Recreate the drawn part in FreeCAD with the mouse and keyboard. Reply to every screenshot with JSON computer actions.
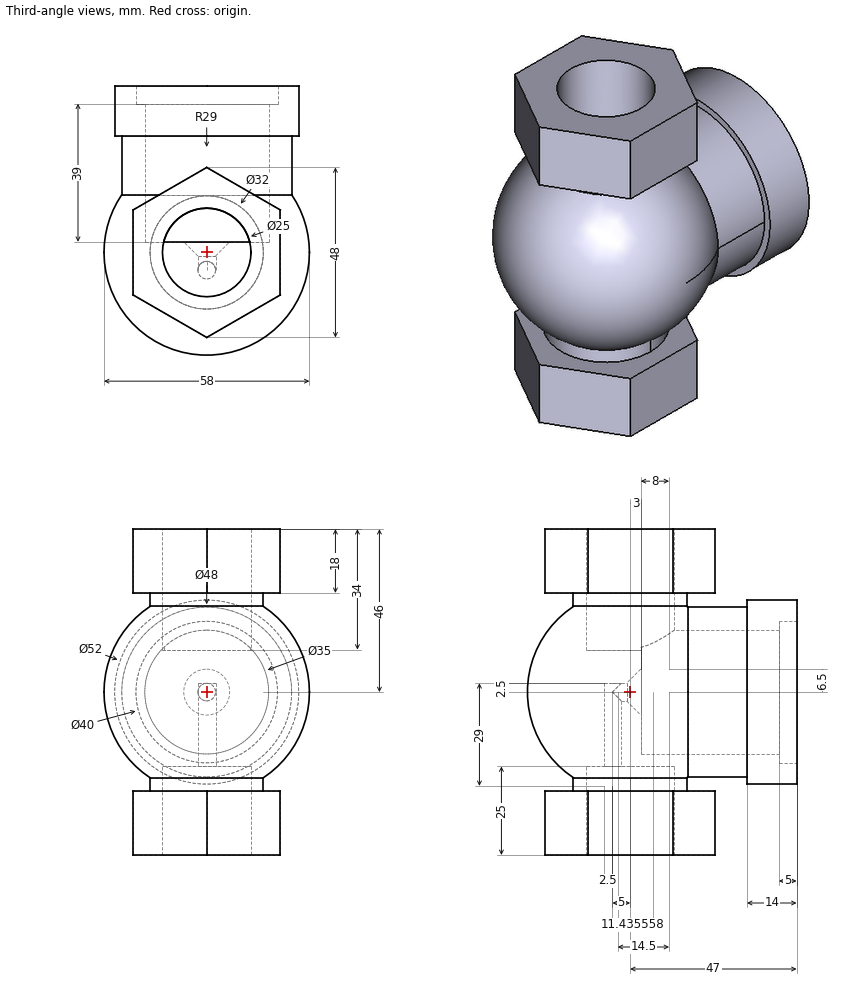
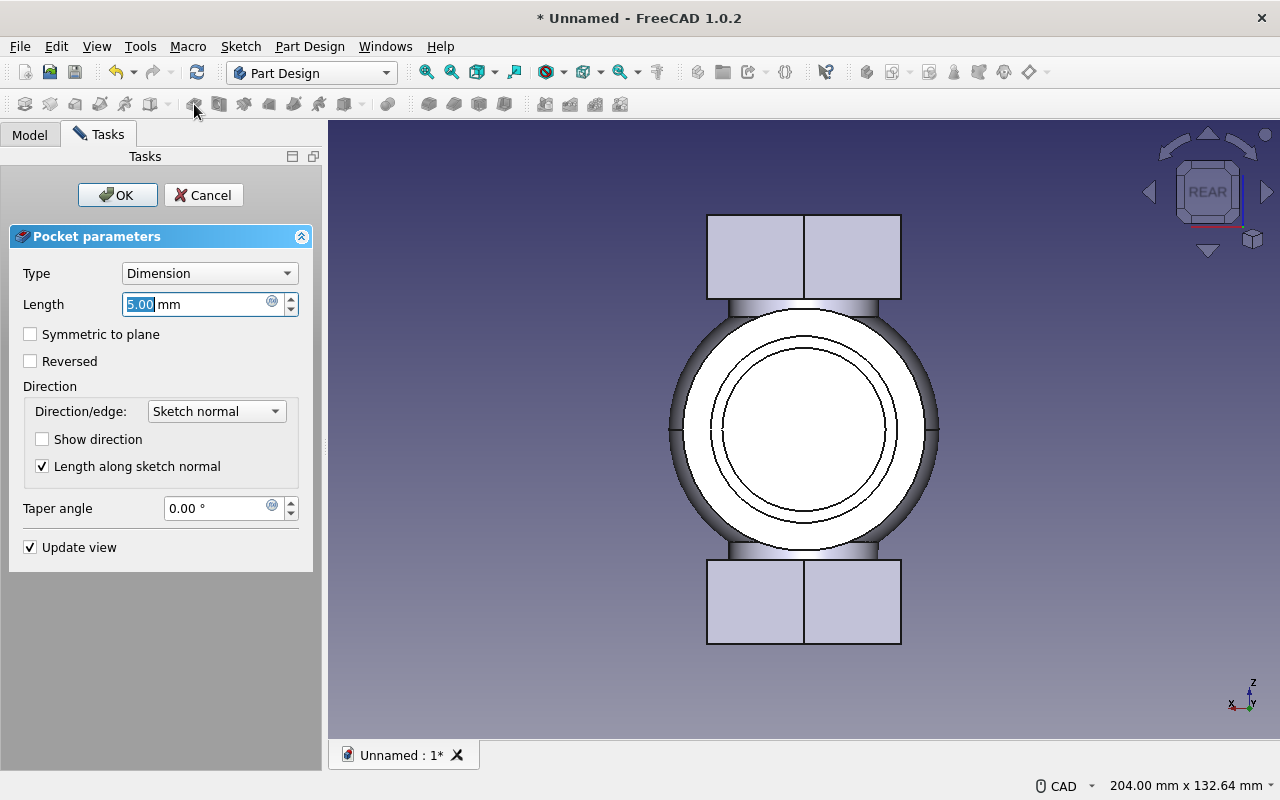
{"action": "type", "text": "39"}
{"action": "key", "text": "Tab"}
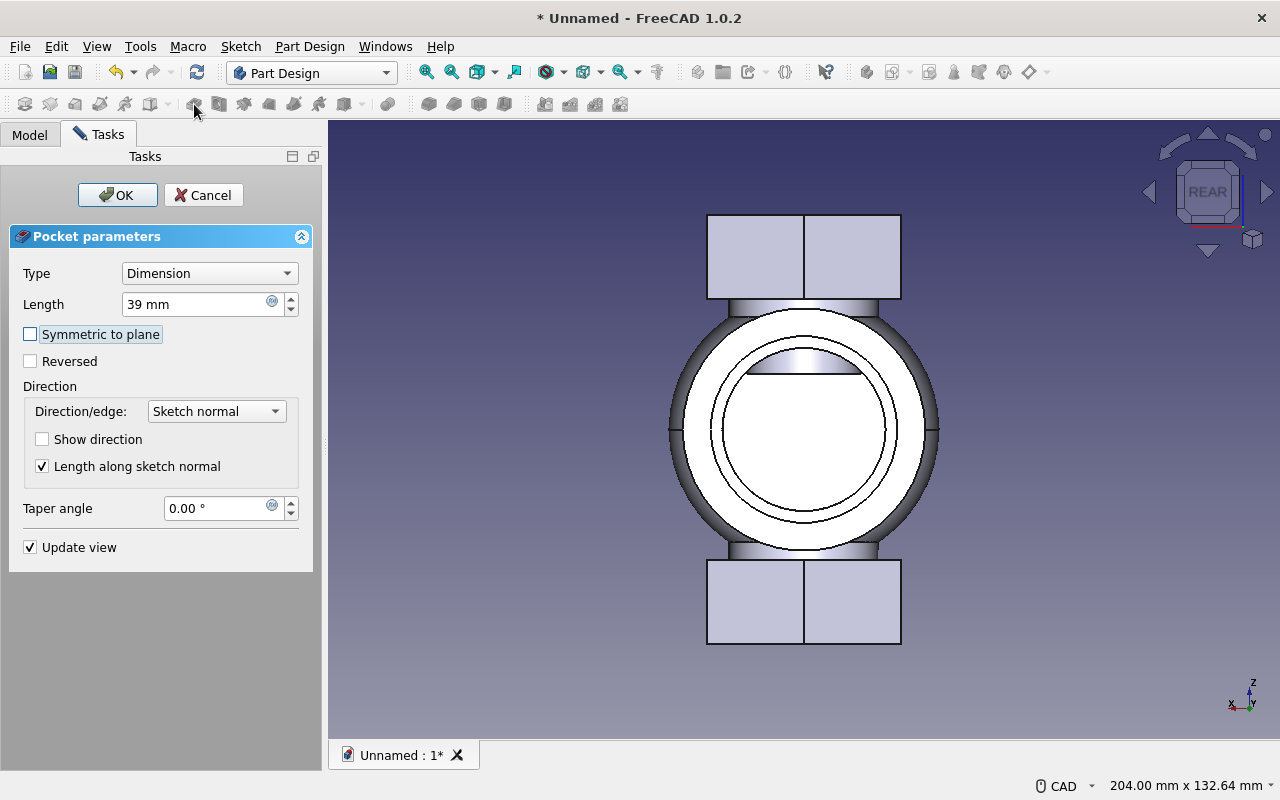
{"action": "left_click", "coordinate": [118, 195]}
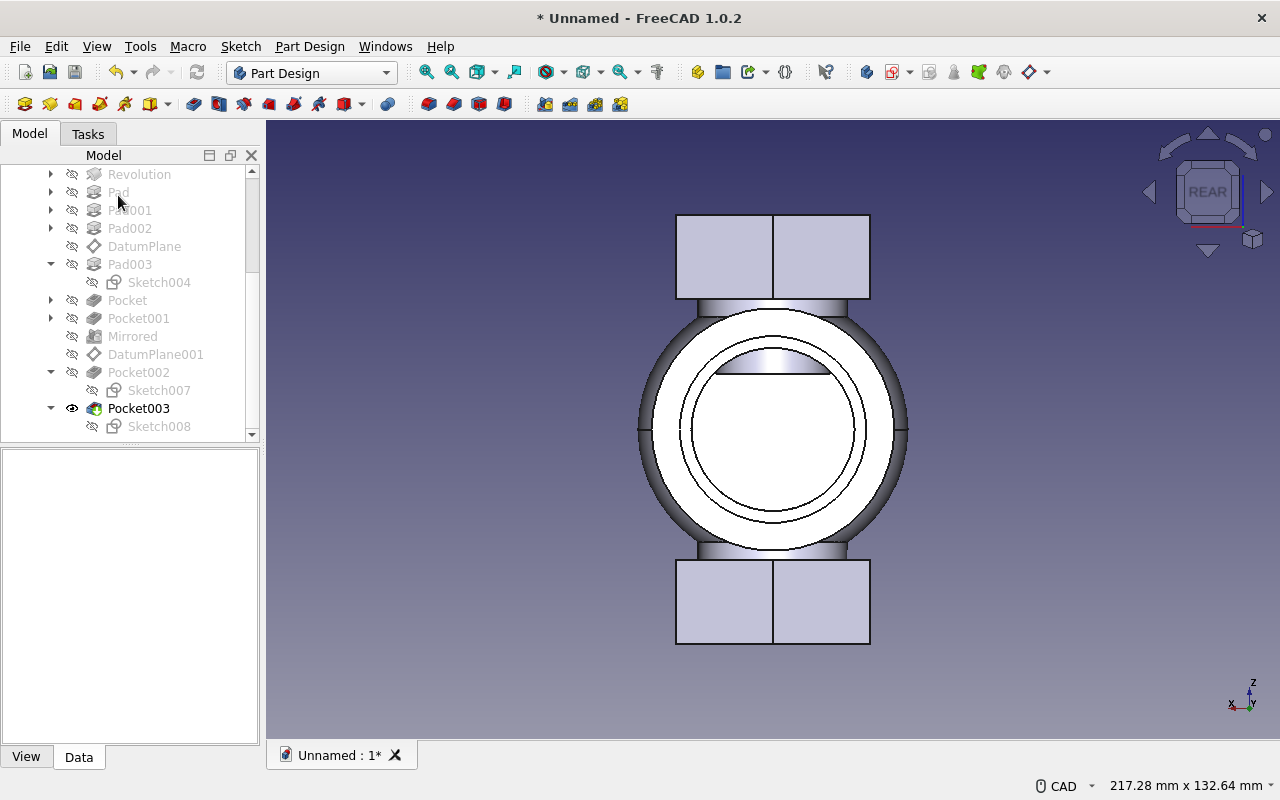
{"action": "left_click", "coordinate": [892, 72]}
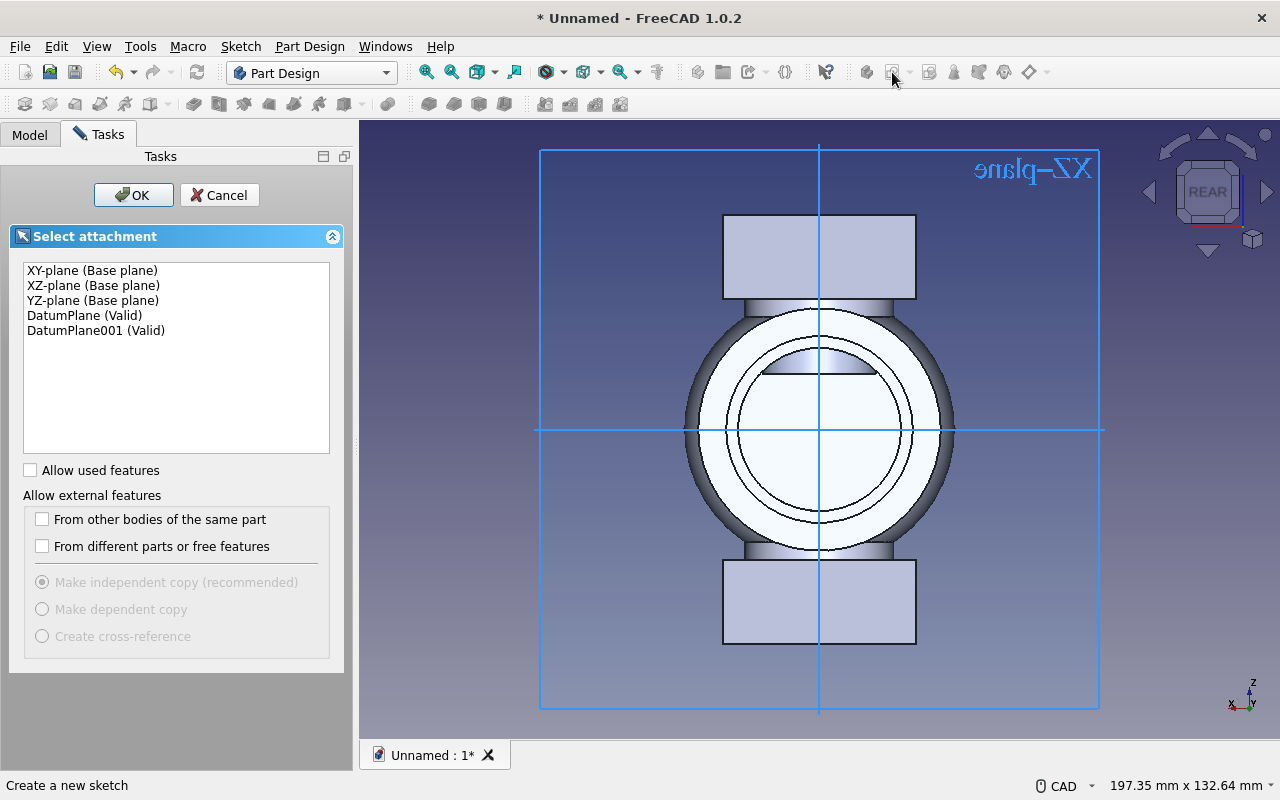
{"action": "left_click", "coordinate": [84, 300]}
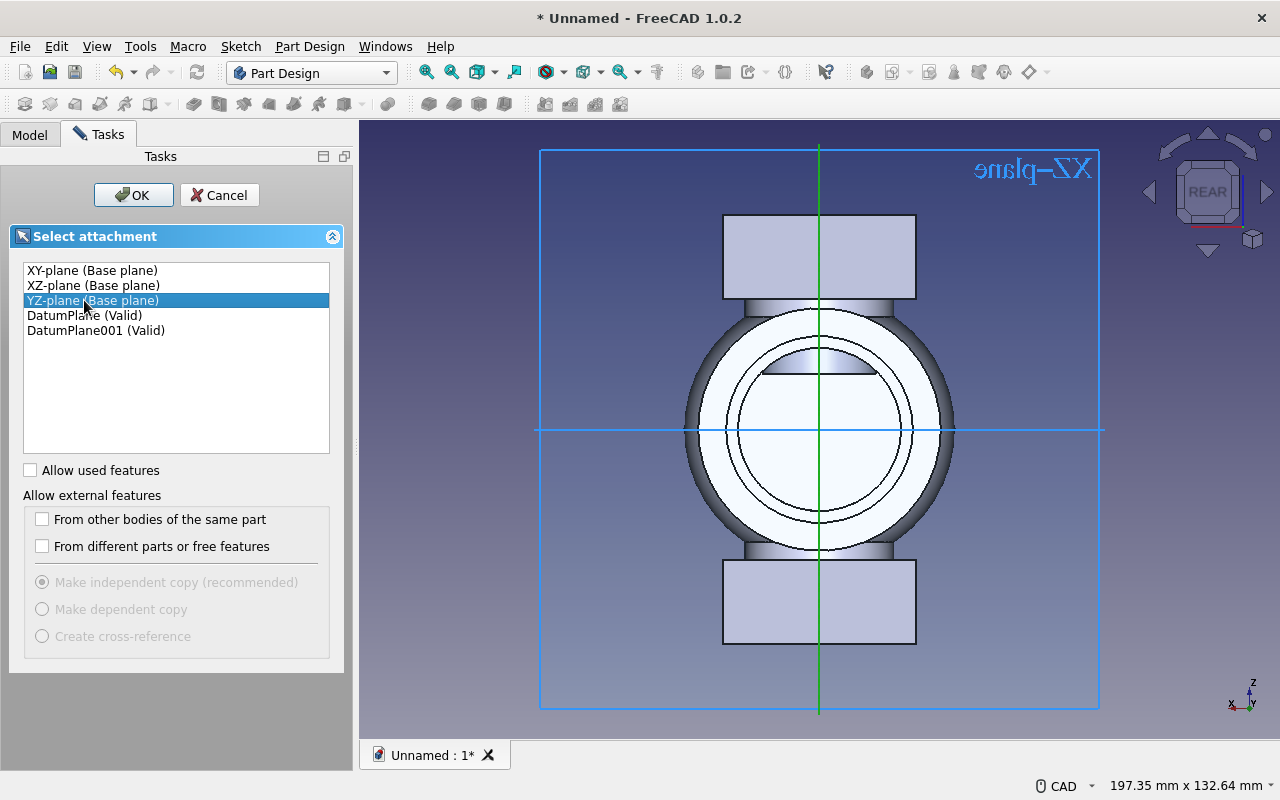
{"action": "left_click", "coordinate": [134, 195]}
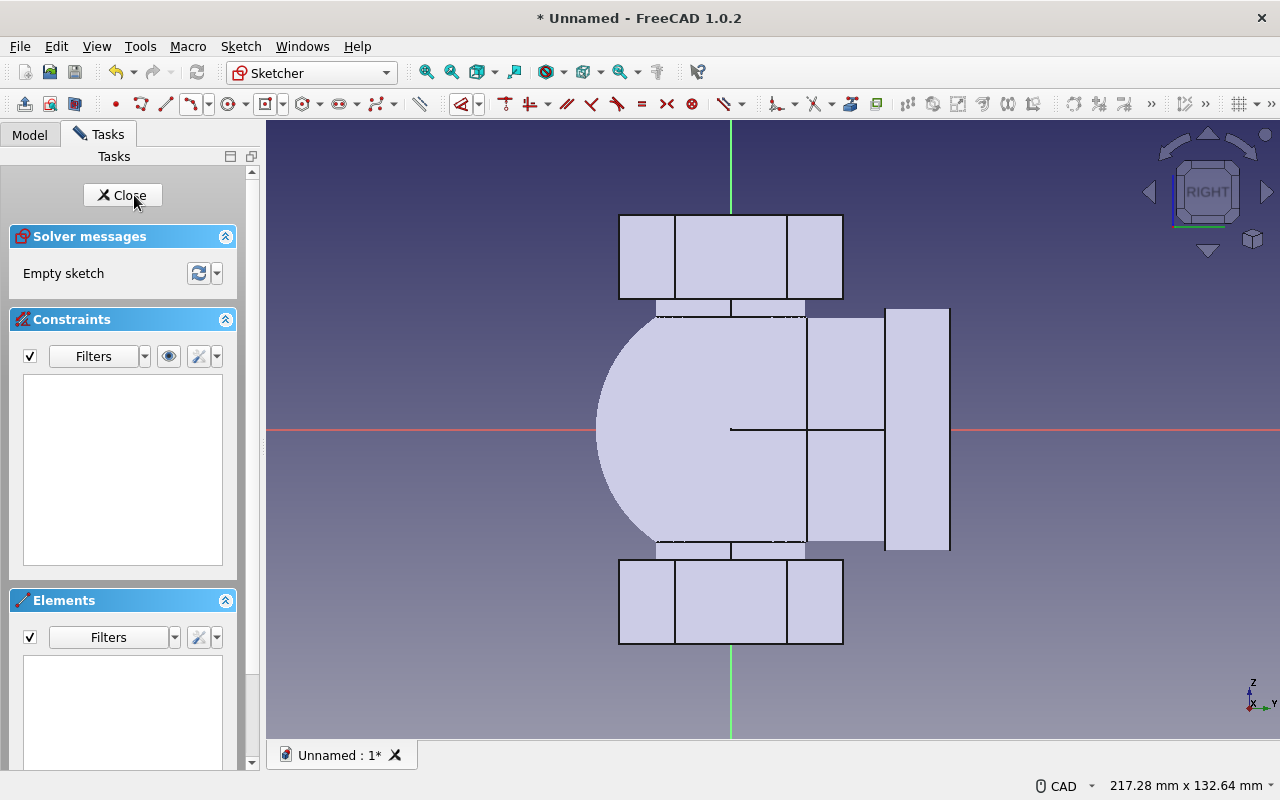
{"action": "left_click", "coordinate": [75, 104]}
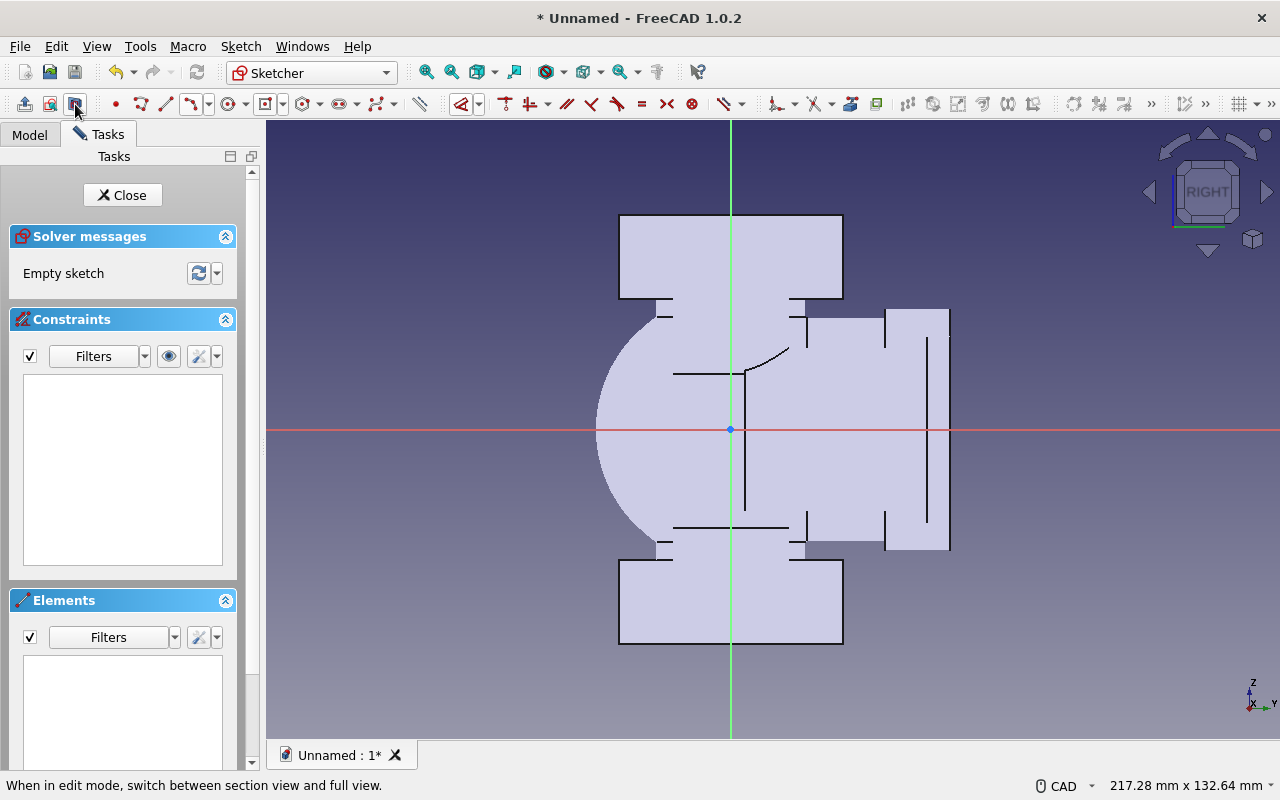
{"action": "scroll", "coordinate": [754, 412], "scroll_direction": "up", "scroll_amount": 11}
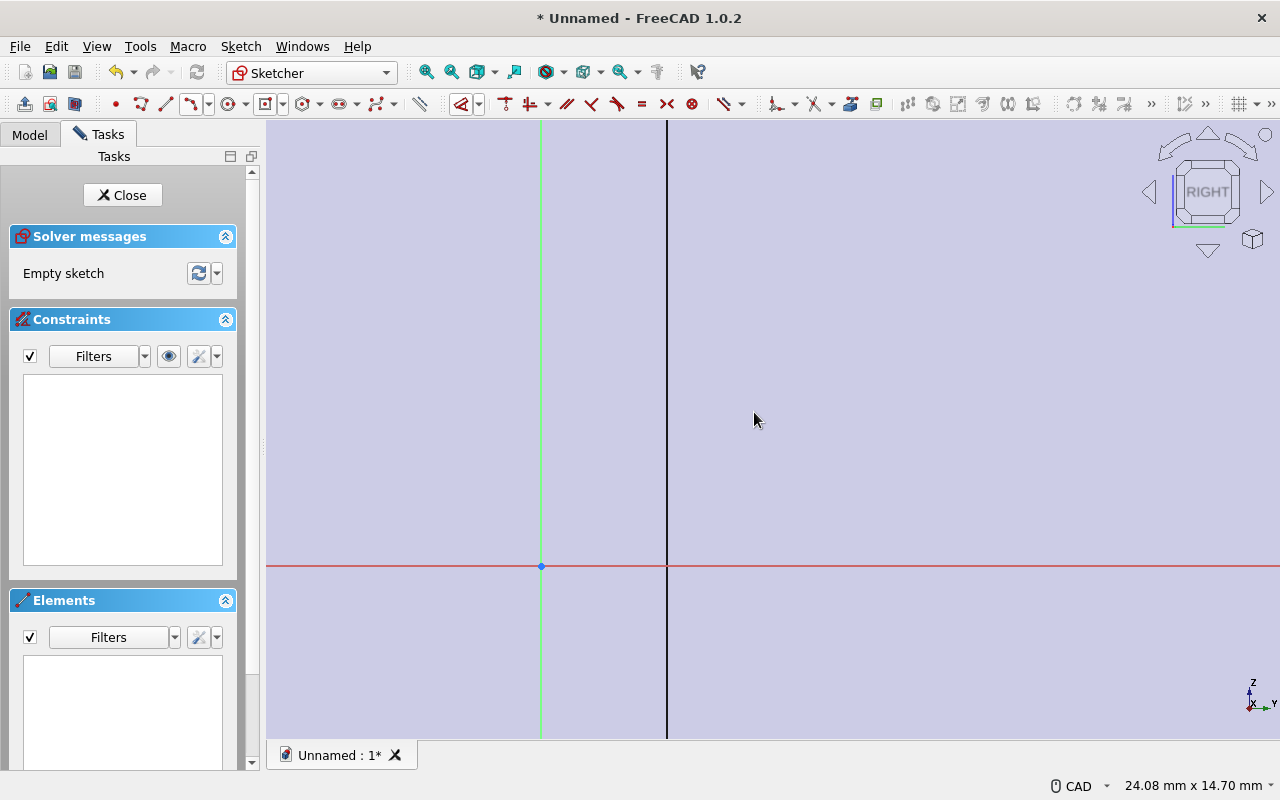
{"action": "left_click", "coordinate": [141, 104]}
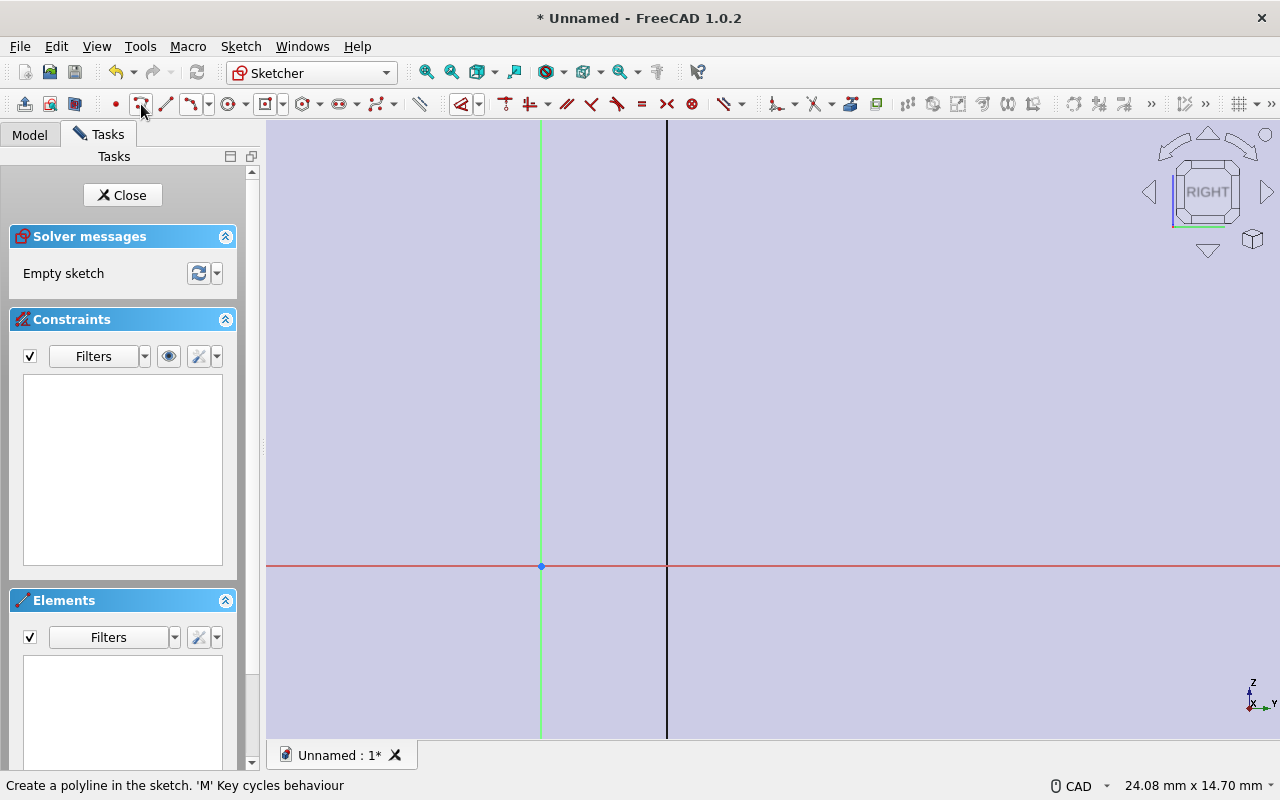
{"action": "left_click", "coordinate": [394, 566]}
{"action": "left_click", "coordinate": [1004, 557]}
{"action": "left_click", "coordinate": [1004, 292]}
{"action": "left_click", "coordinate": [667, 292]}
{"action": "left_click", "coordinate": [394, 566]}
{"action": "key", "text": "Escape"}
{"action": "key", "text": "Escape"}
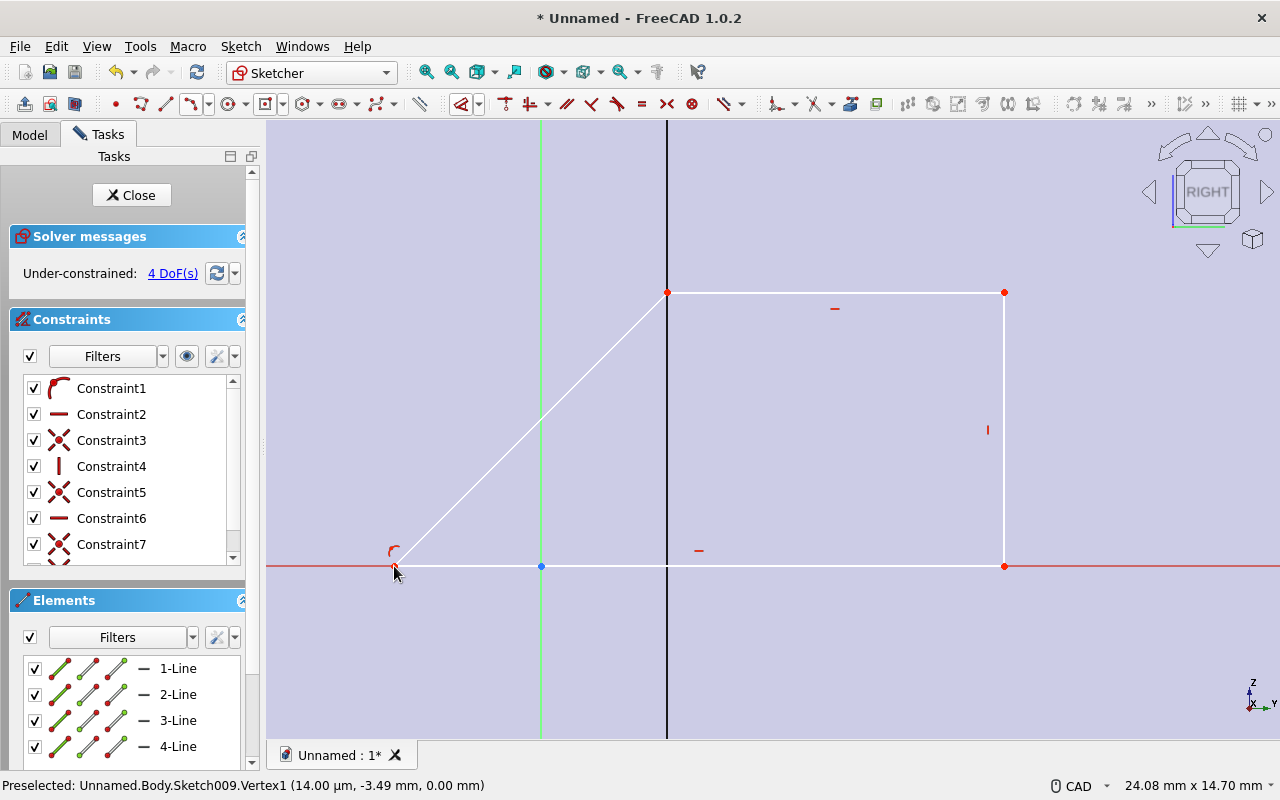
{"action": "left_click", "coordinate": [903, 293]}